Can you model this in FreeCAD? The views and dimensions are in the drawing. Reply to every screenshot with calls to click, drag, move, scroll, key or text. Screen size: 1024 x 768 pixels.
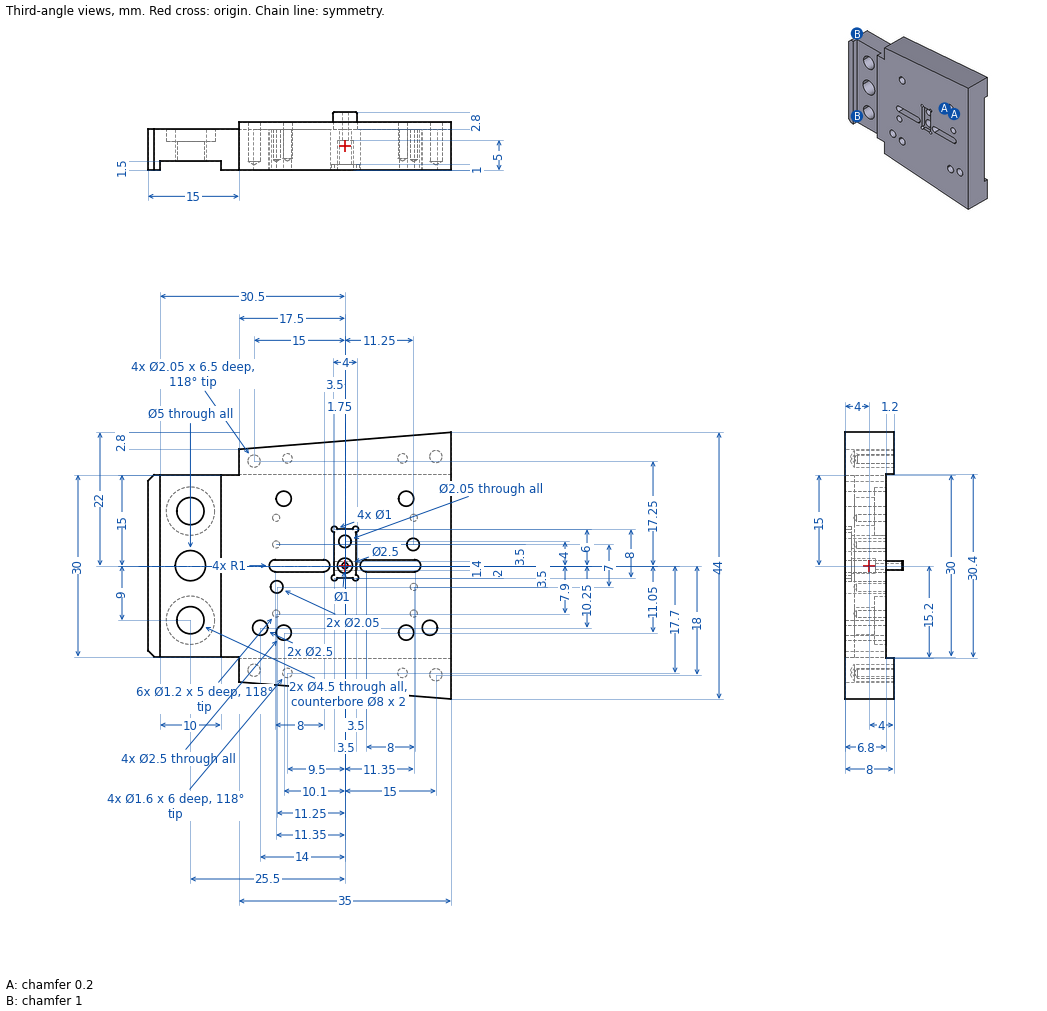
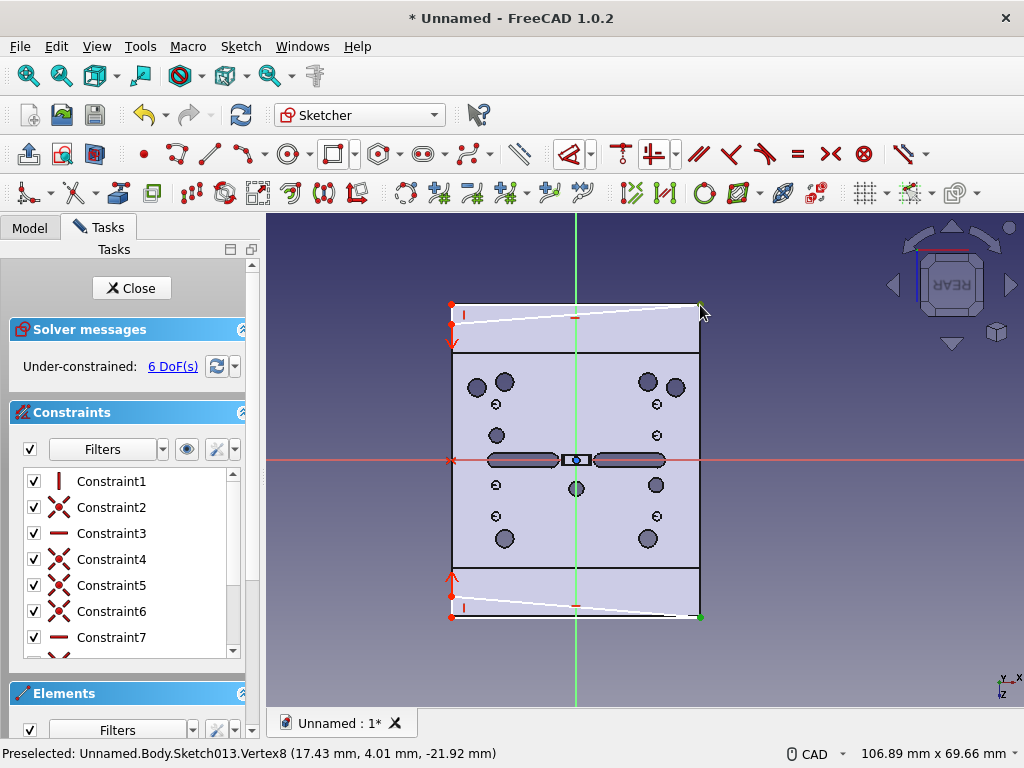
click(334, 460)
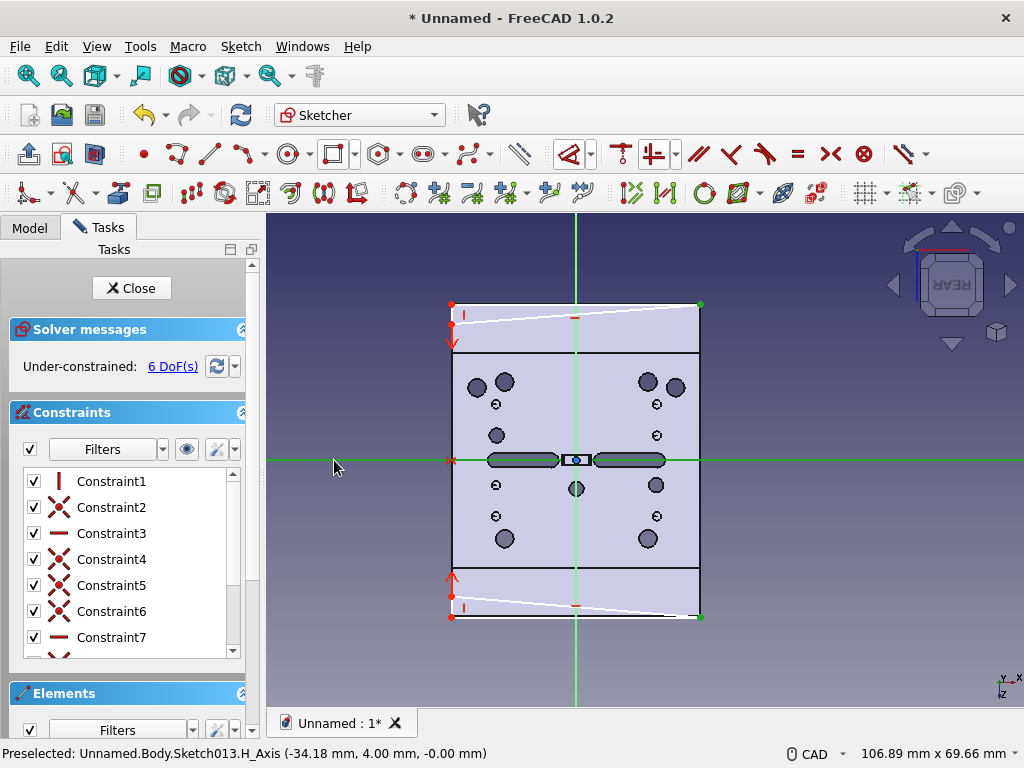
click(831, 154)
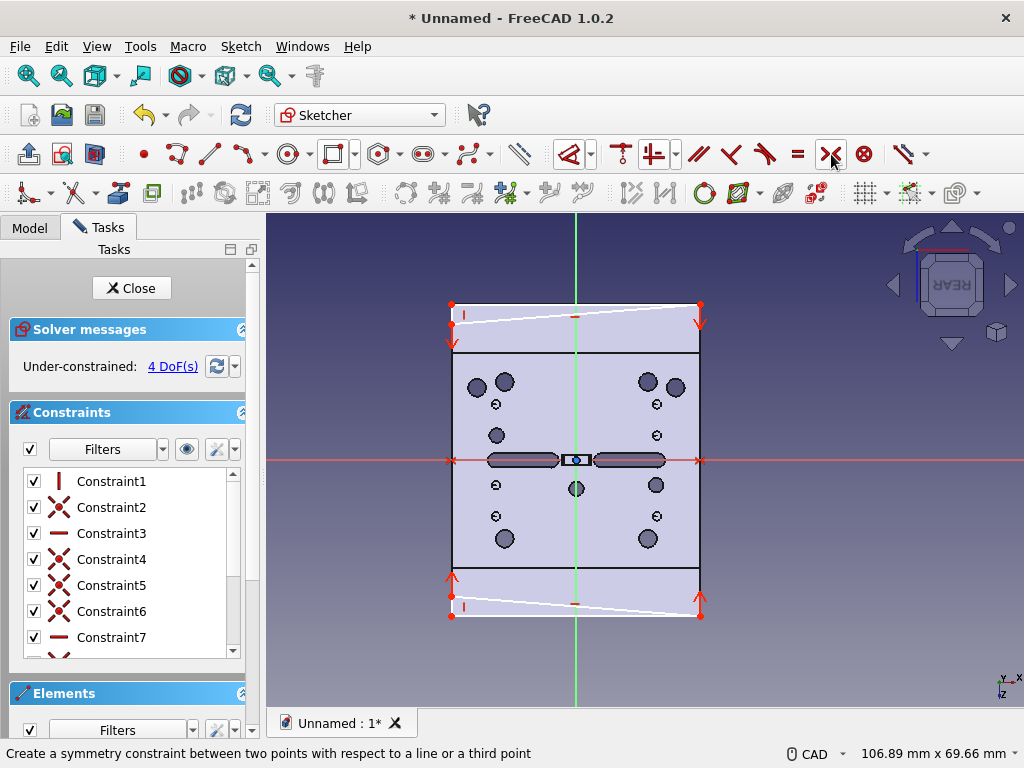
click(526, 616)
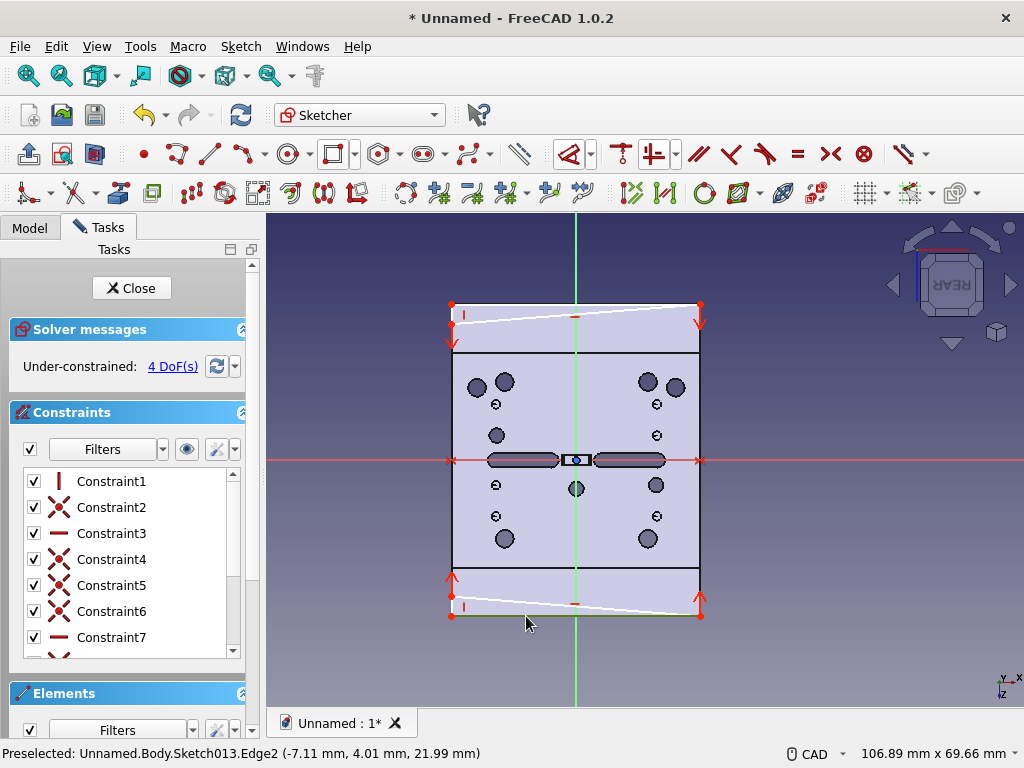
click(590, 154)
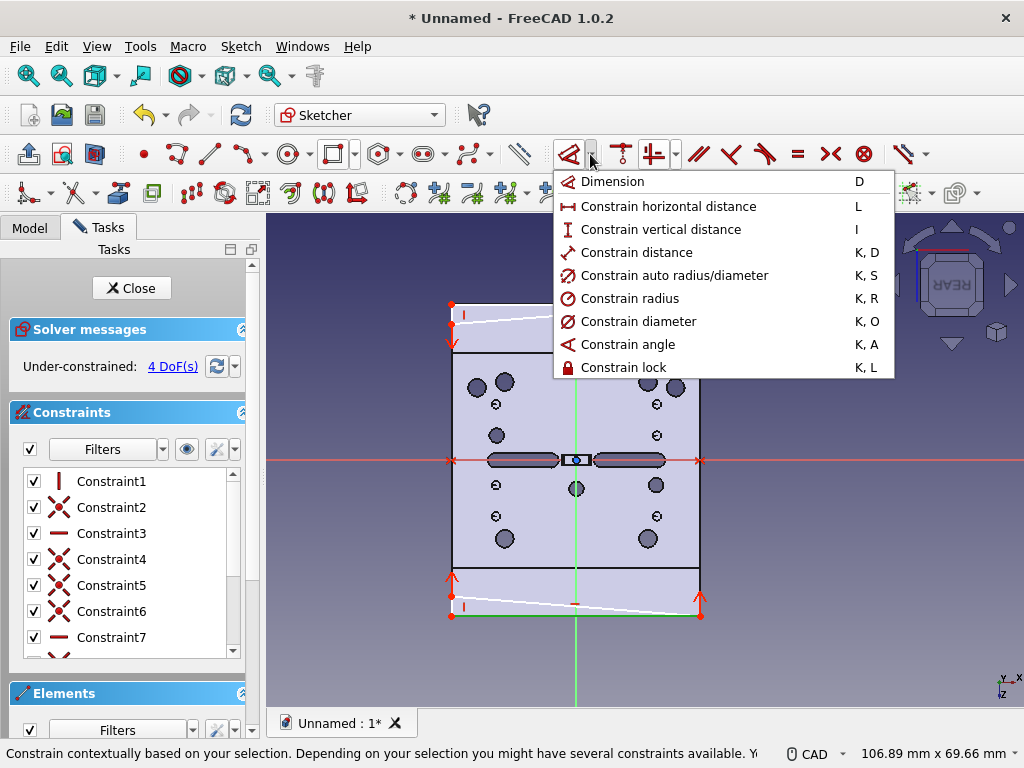
click(724, 206)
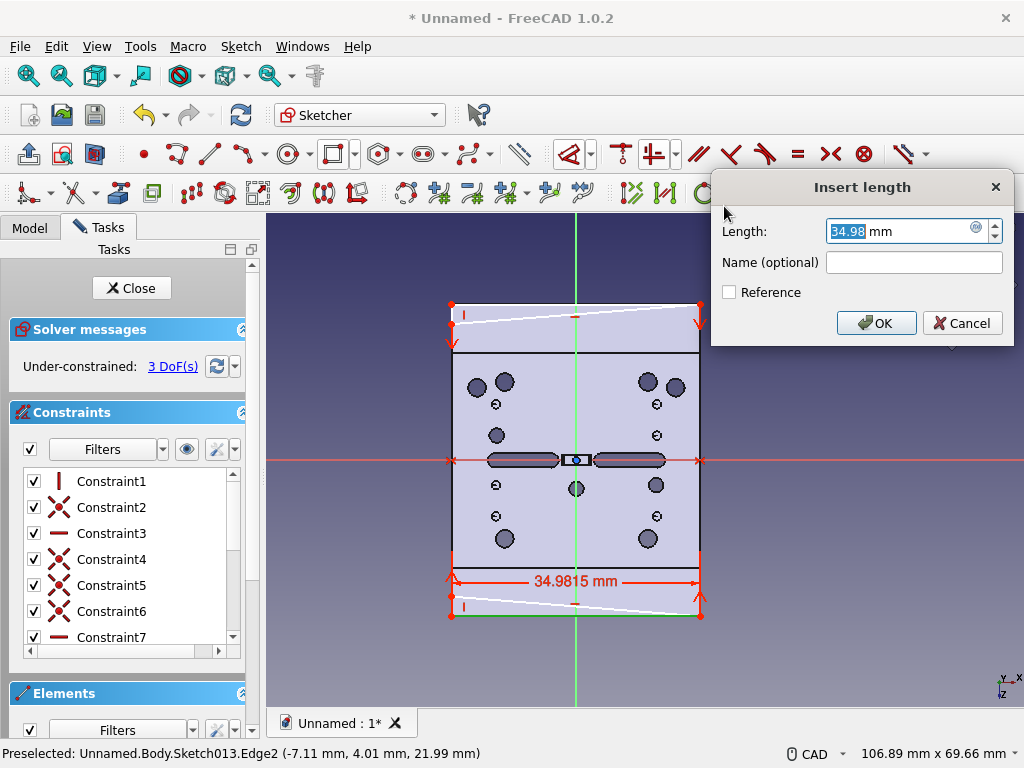
text(35)
key(Return)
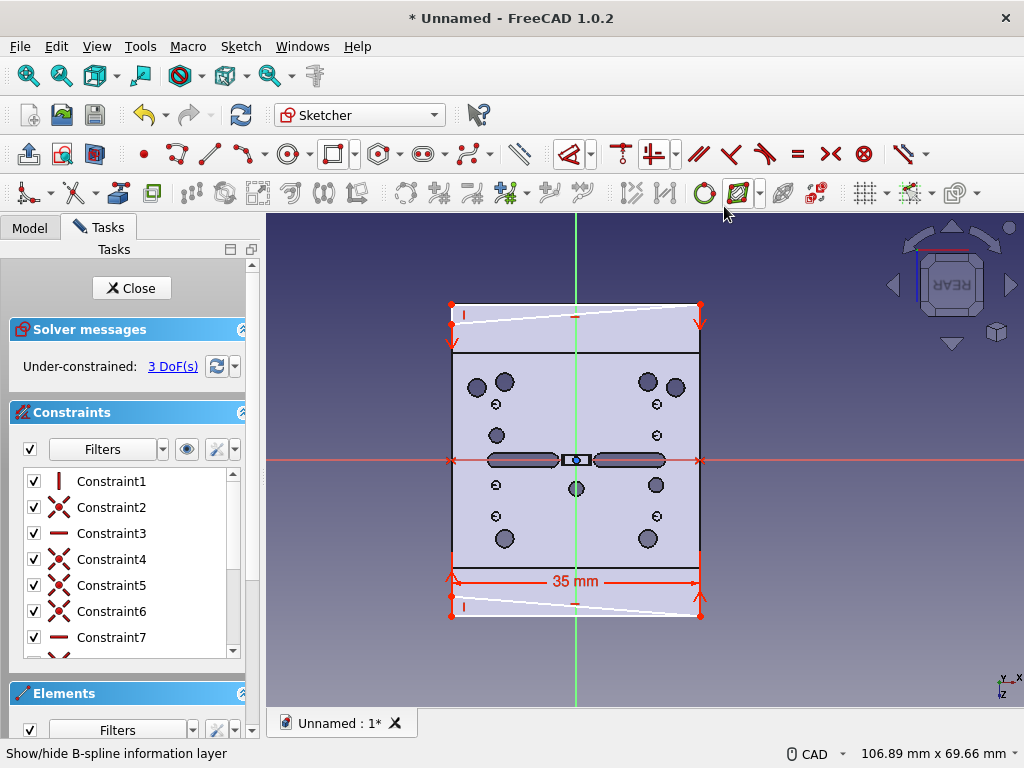
scroll(452, 606, up, 4)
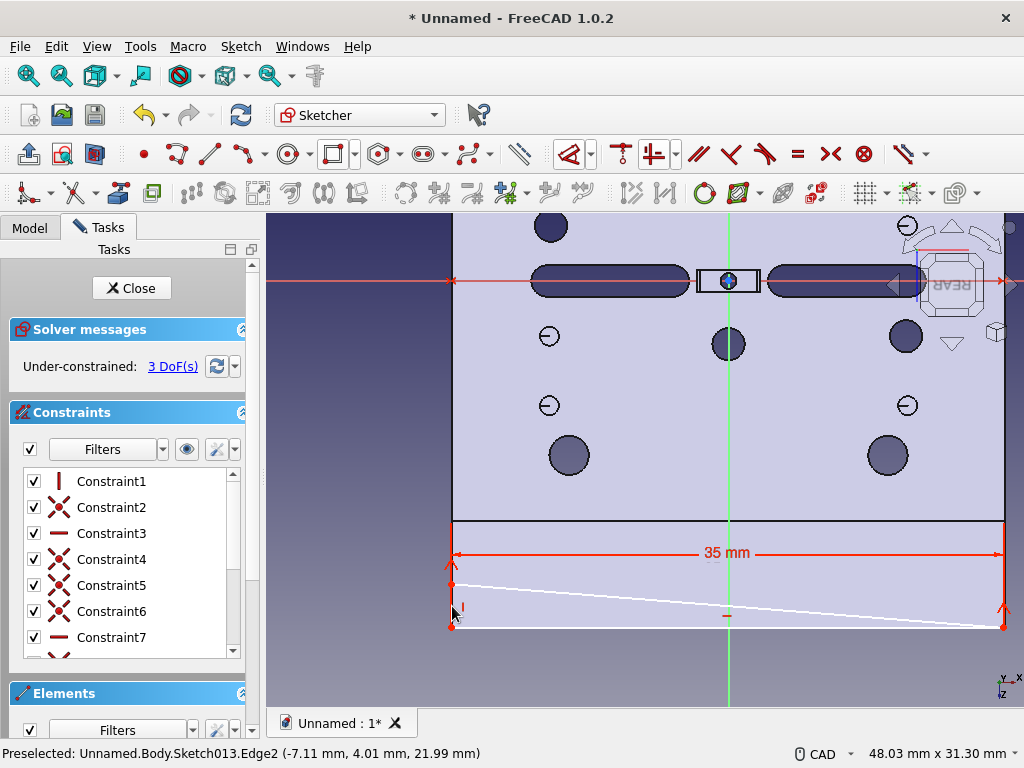
click(451, 606)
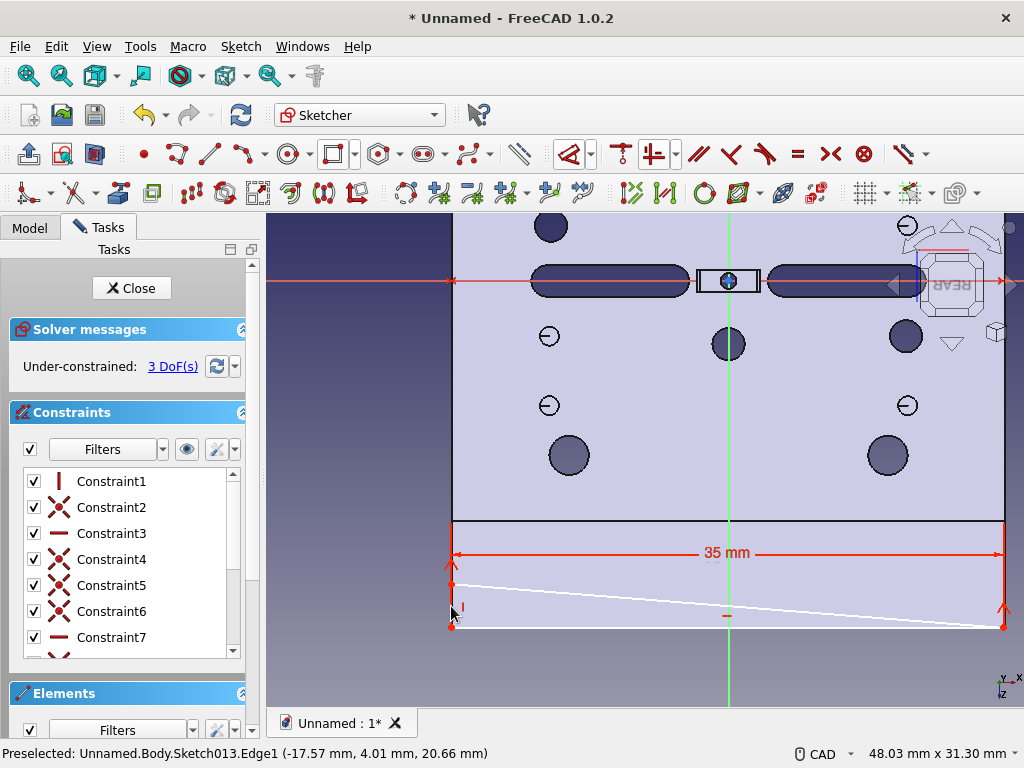
click(590, 154)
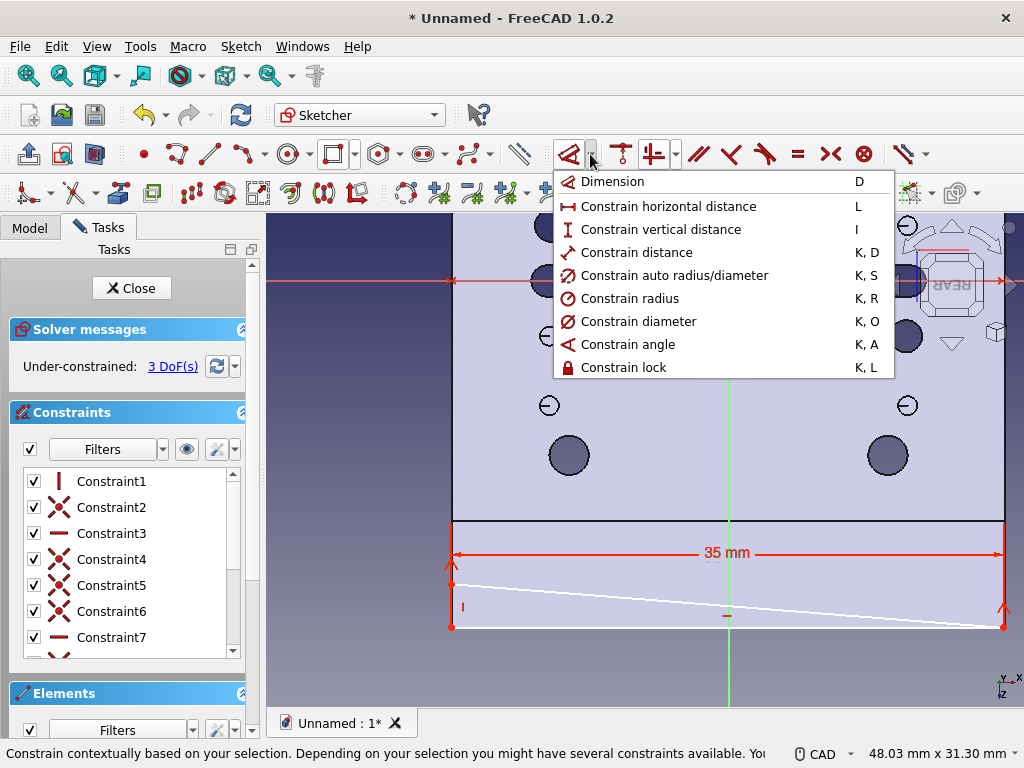
click(724, 230)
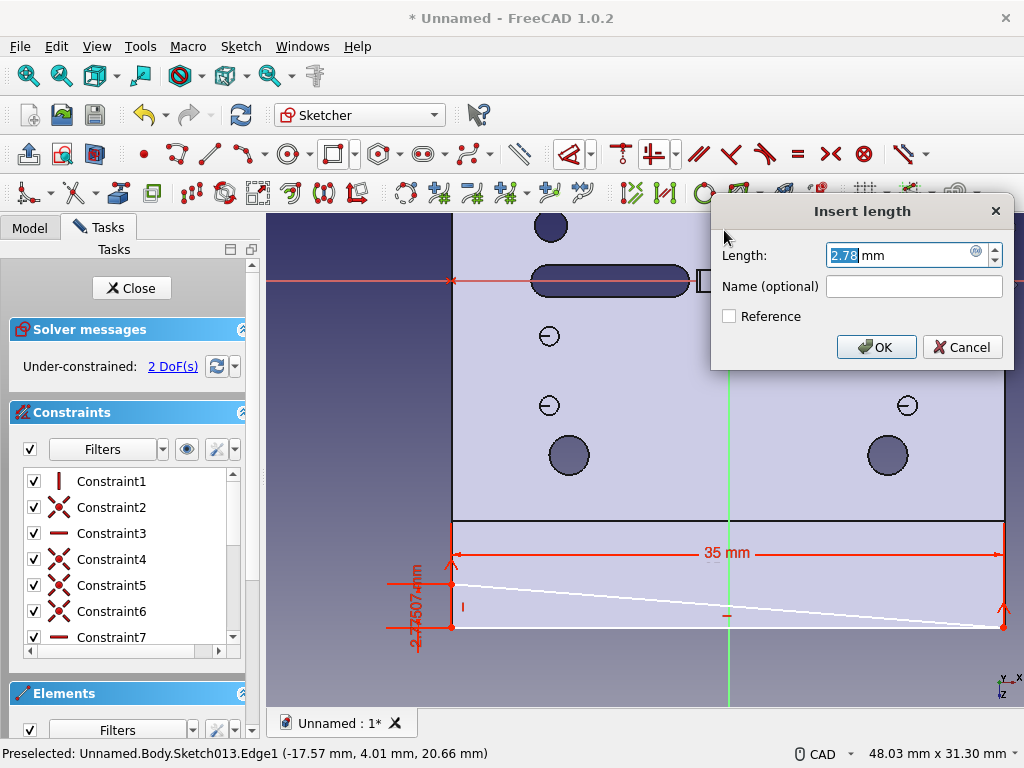
text(2.8)
key(Return)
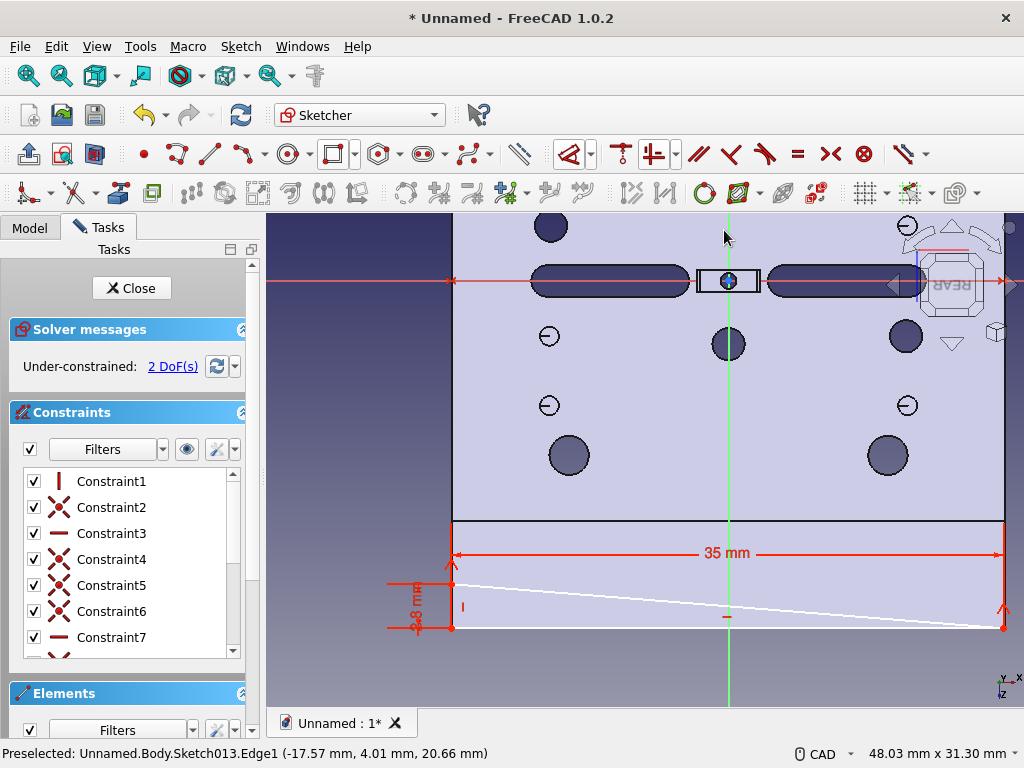
click(451, 628)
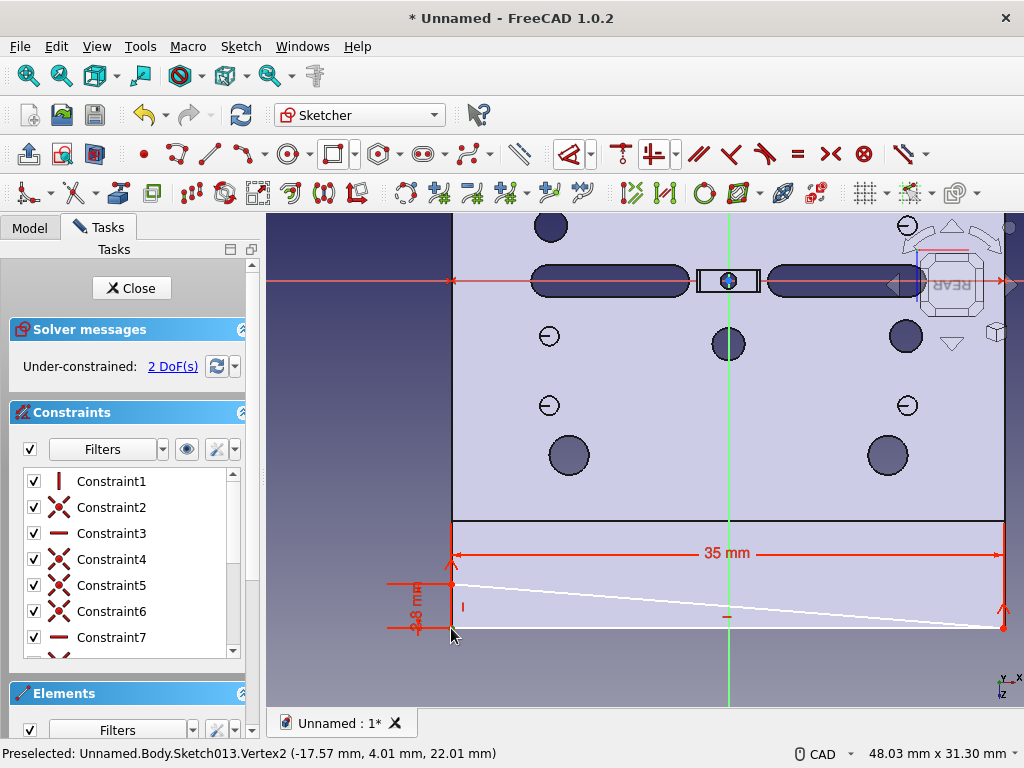
click(590, 154)